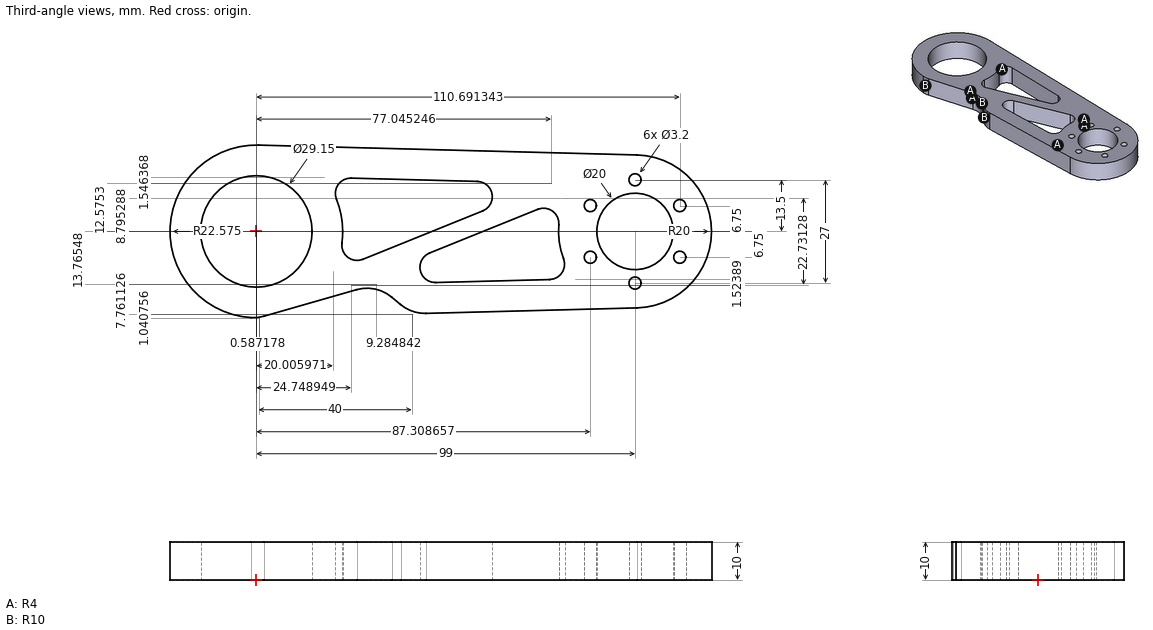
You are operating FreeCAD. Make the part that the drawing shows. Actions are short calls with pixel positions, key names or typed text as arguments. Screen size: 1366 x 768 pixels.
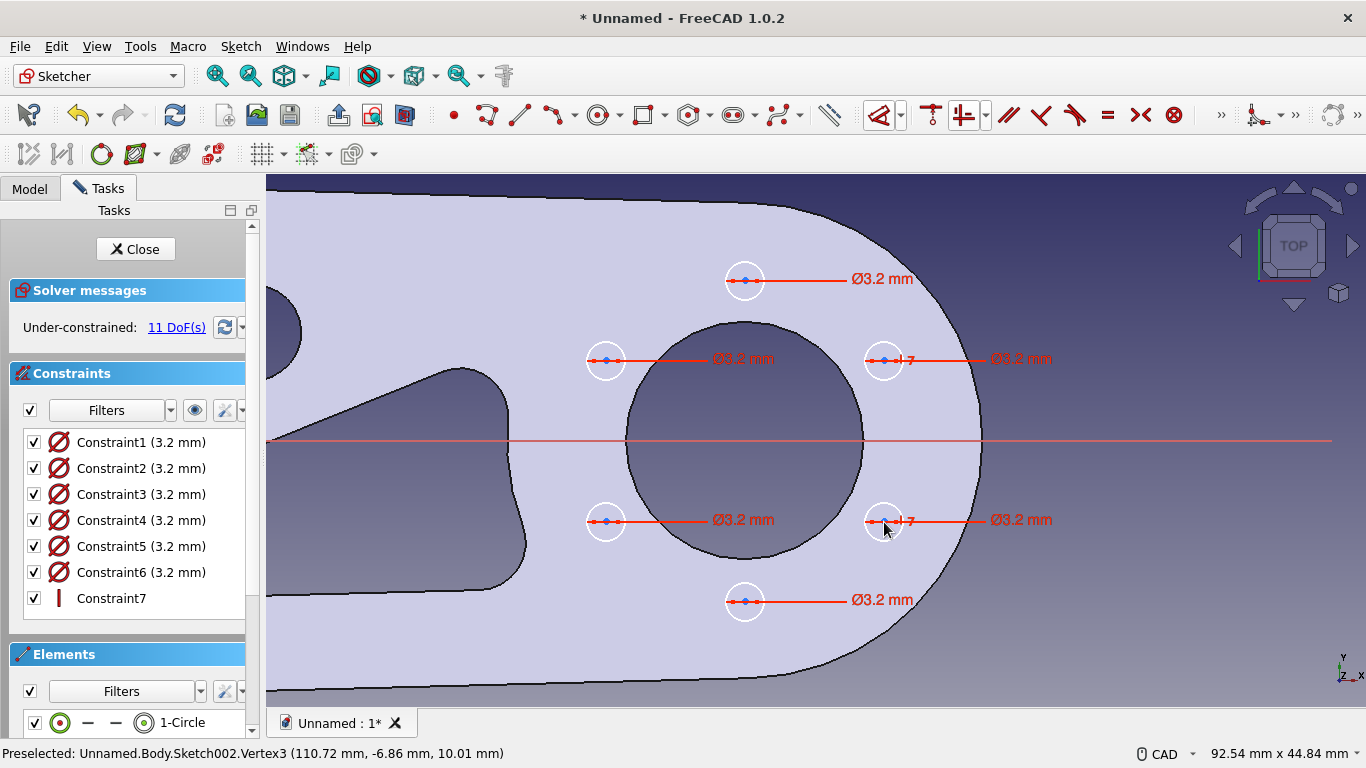
click(745, 281)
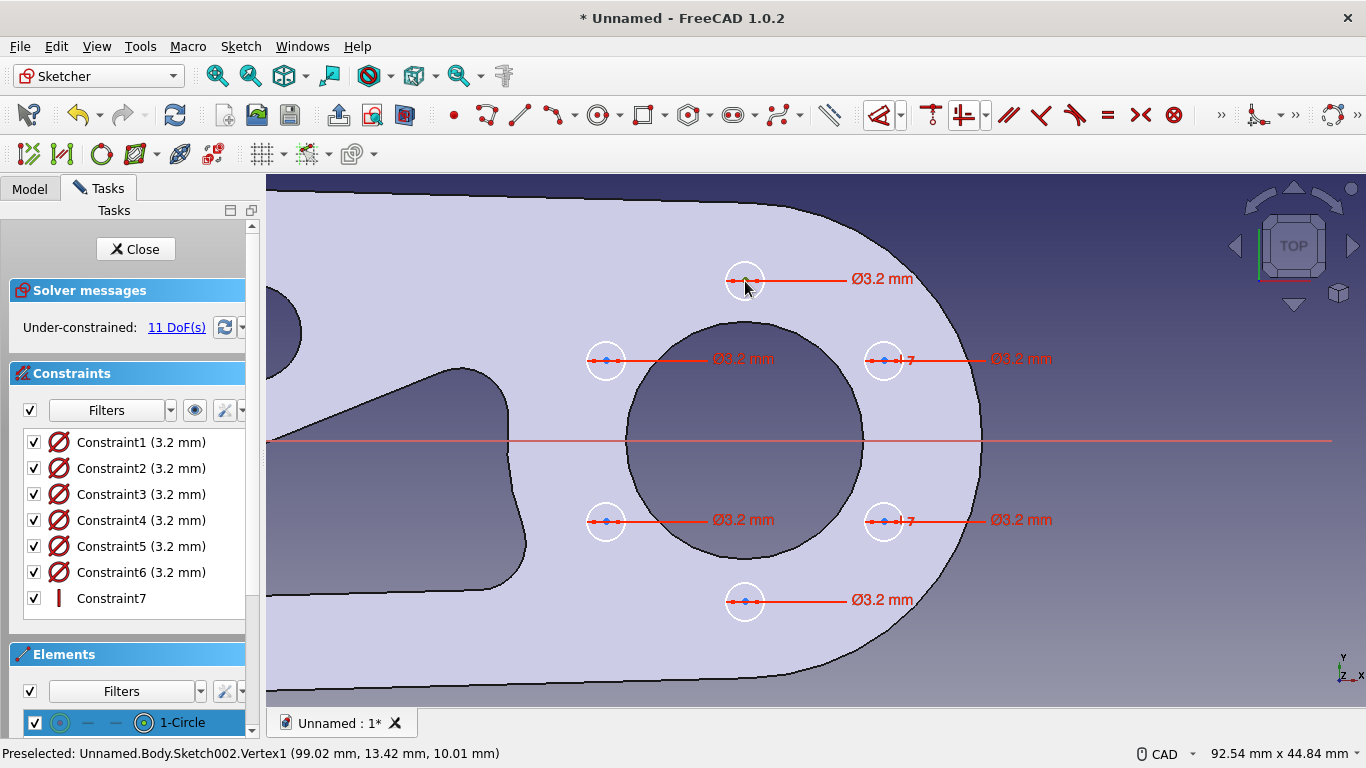
click(745, 602)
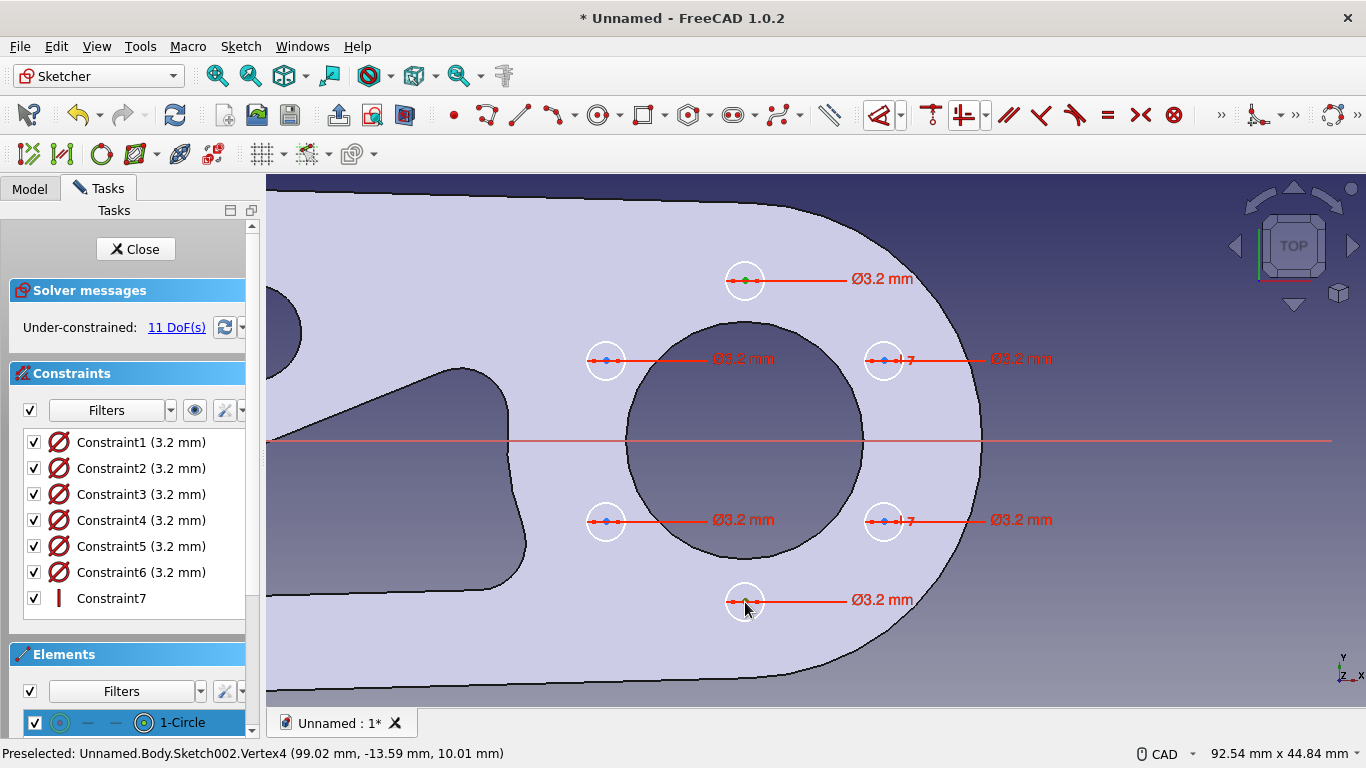
click(986, 116)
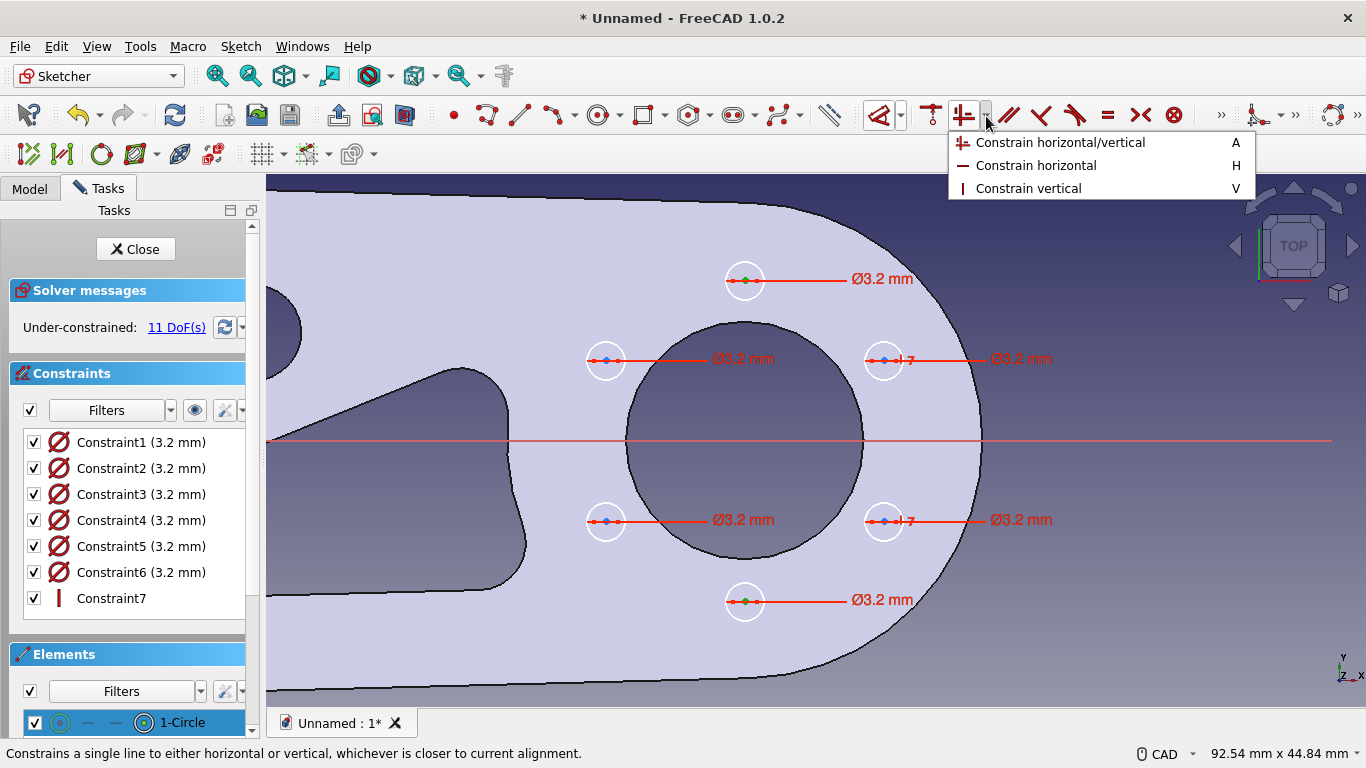
click(1102, 188)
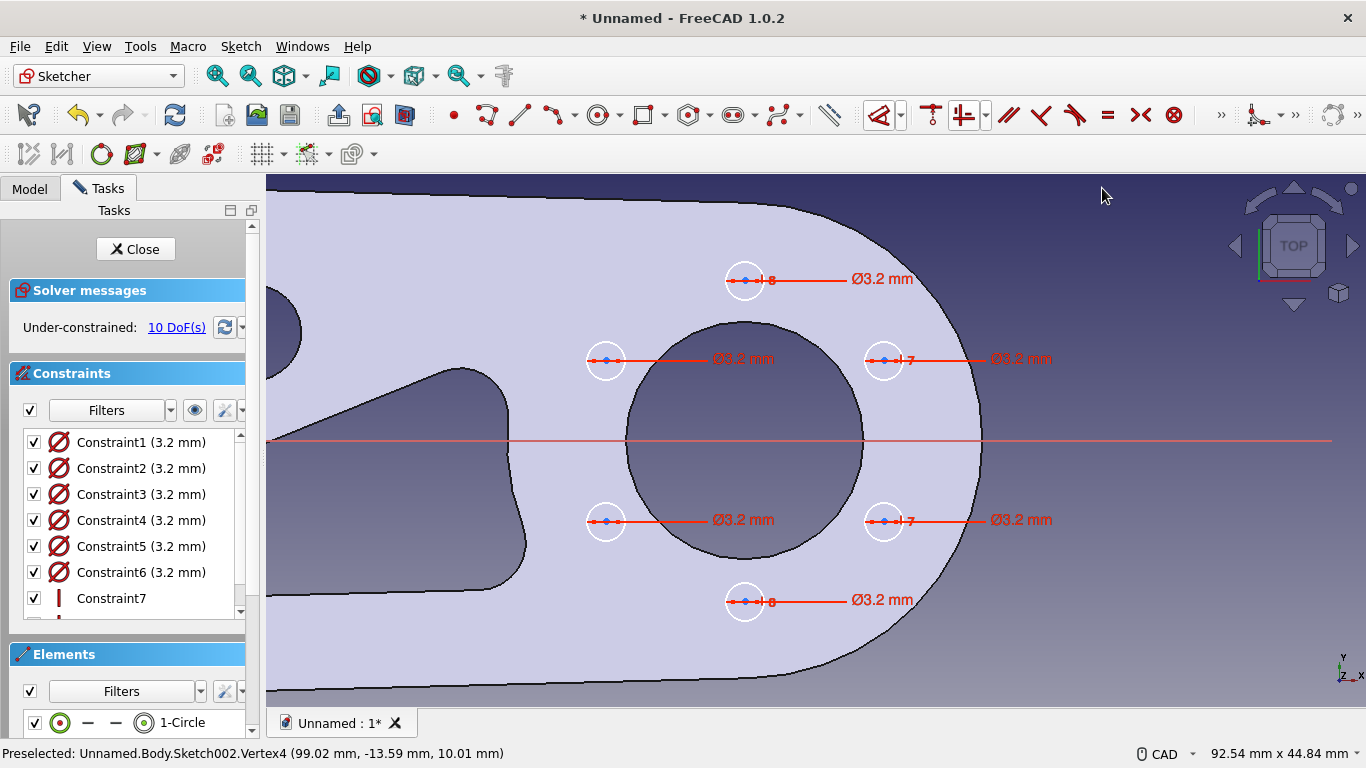
click(884, 522)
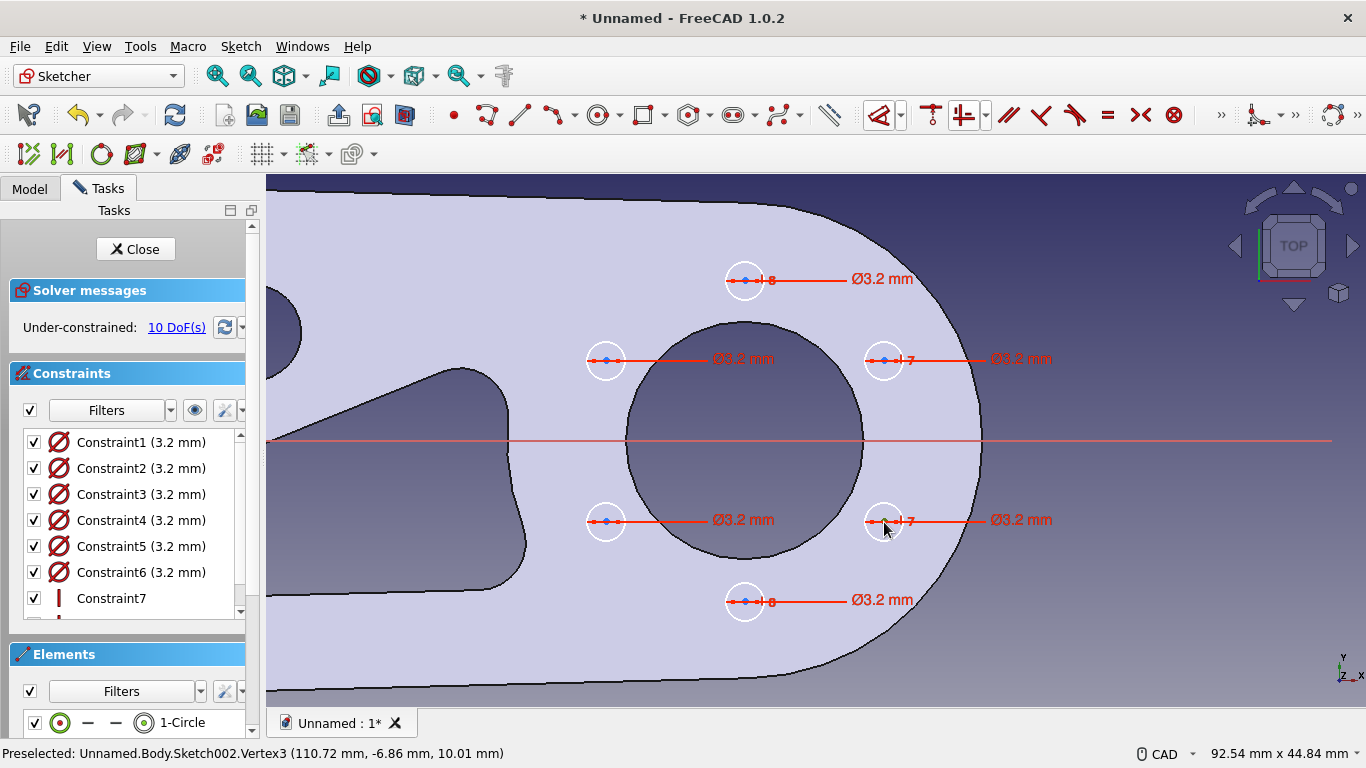
click(606, 522)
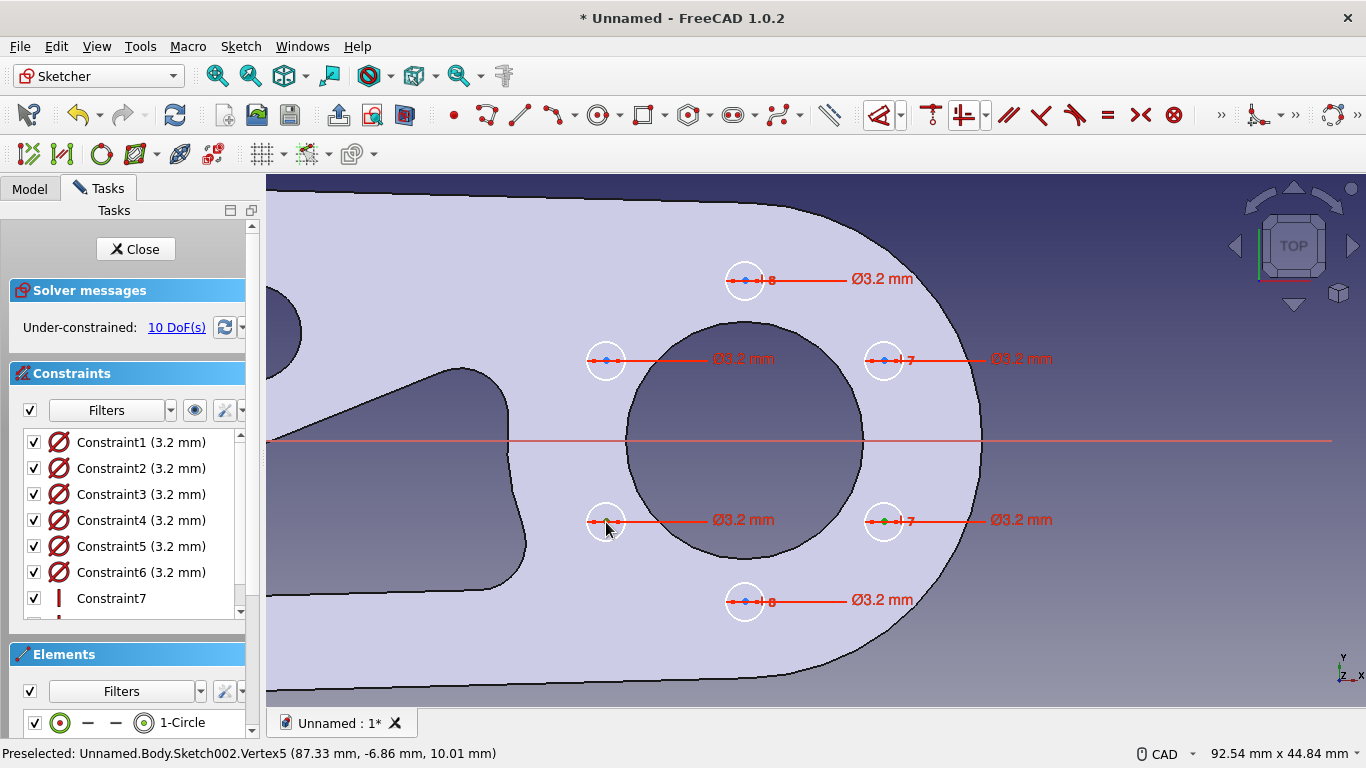
key(h)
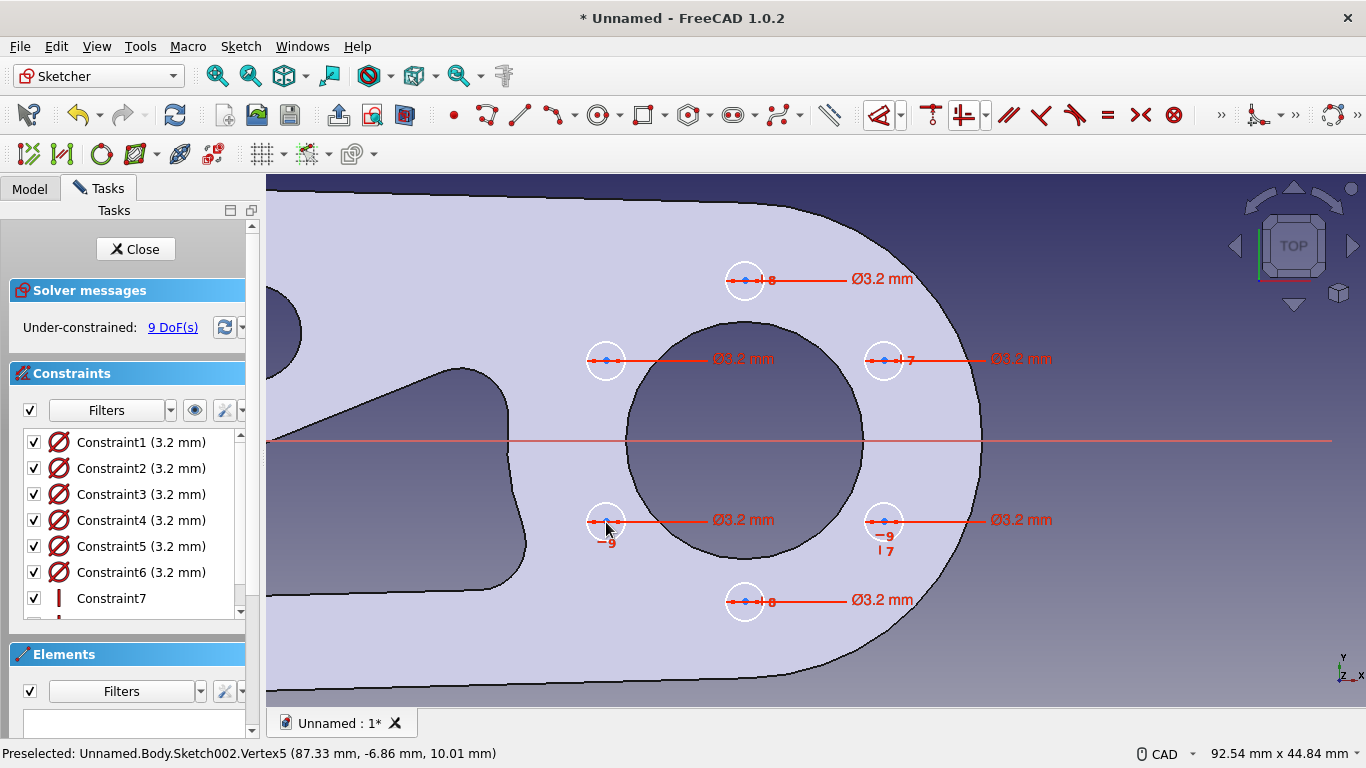
click(606, 522)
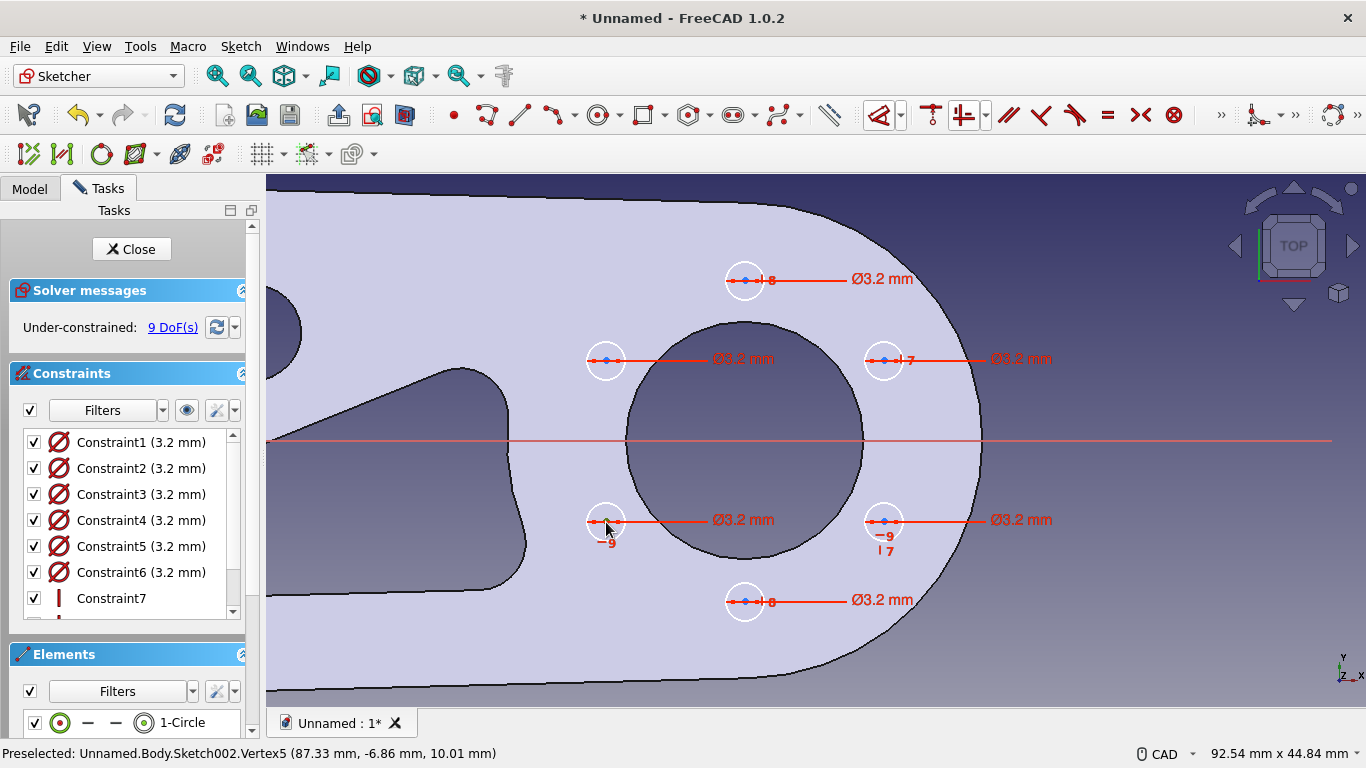
click(606, 361)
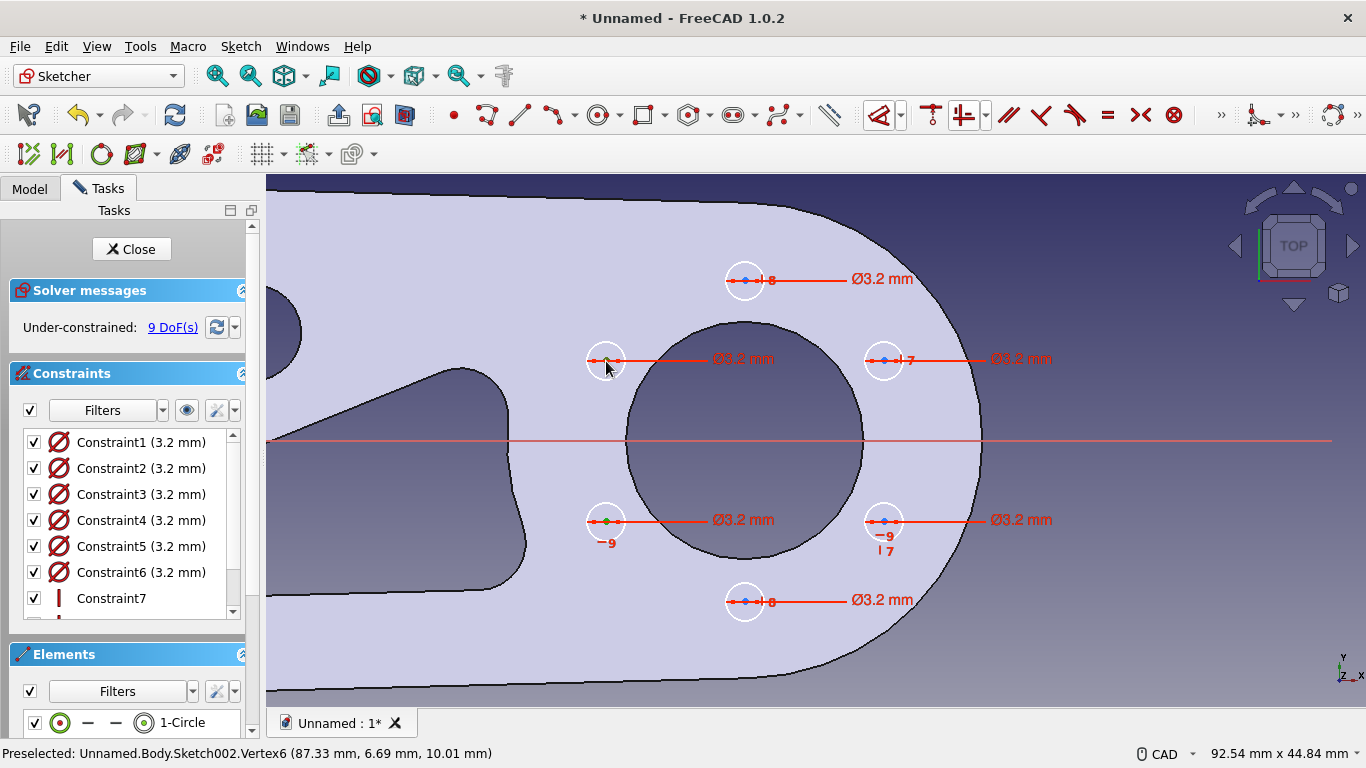
click(986, 116)